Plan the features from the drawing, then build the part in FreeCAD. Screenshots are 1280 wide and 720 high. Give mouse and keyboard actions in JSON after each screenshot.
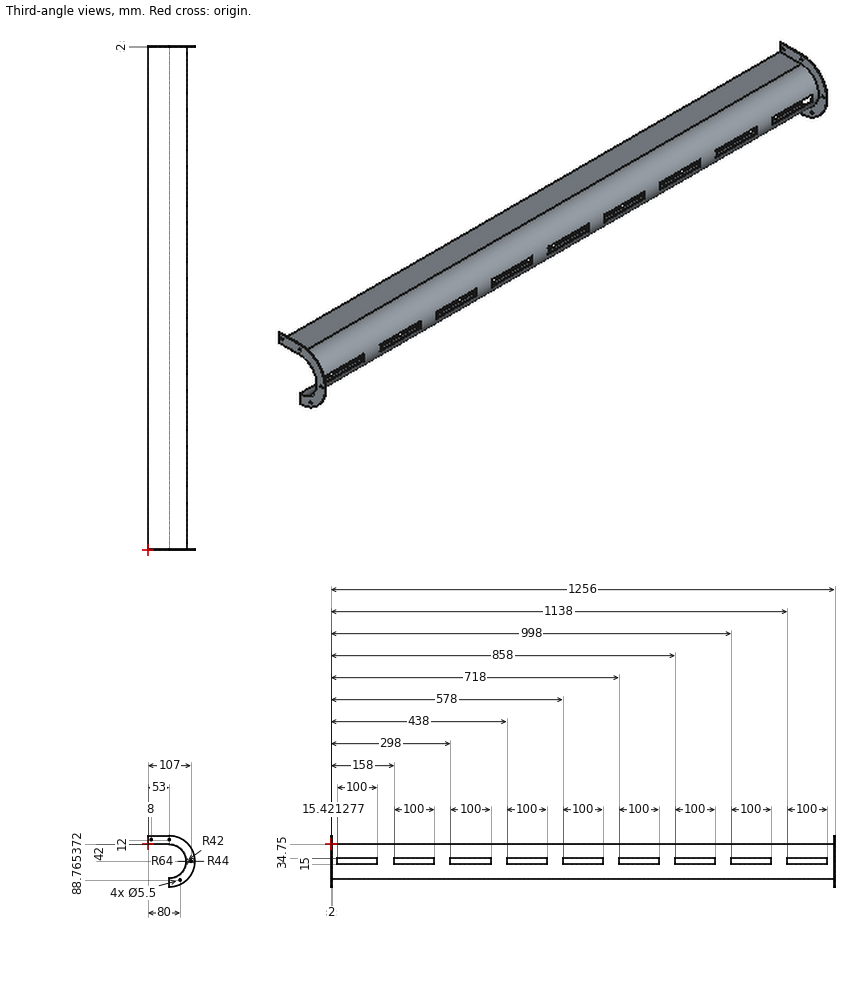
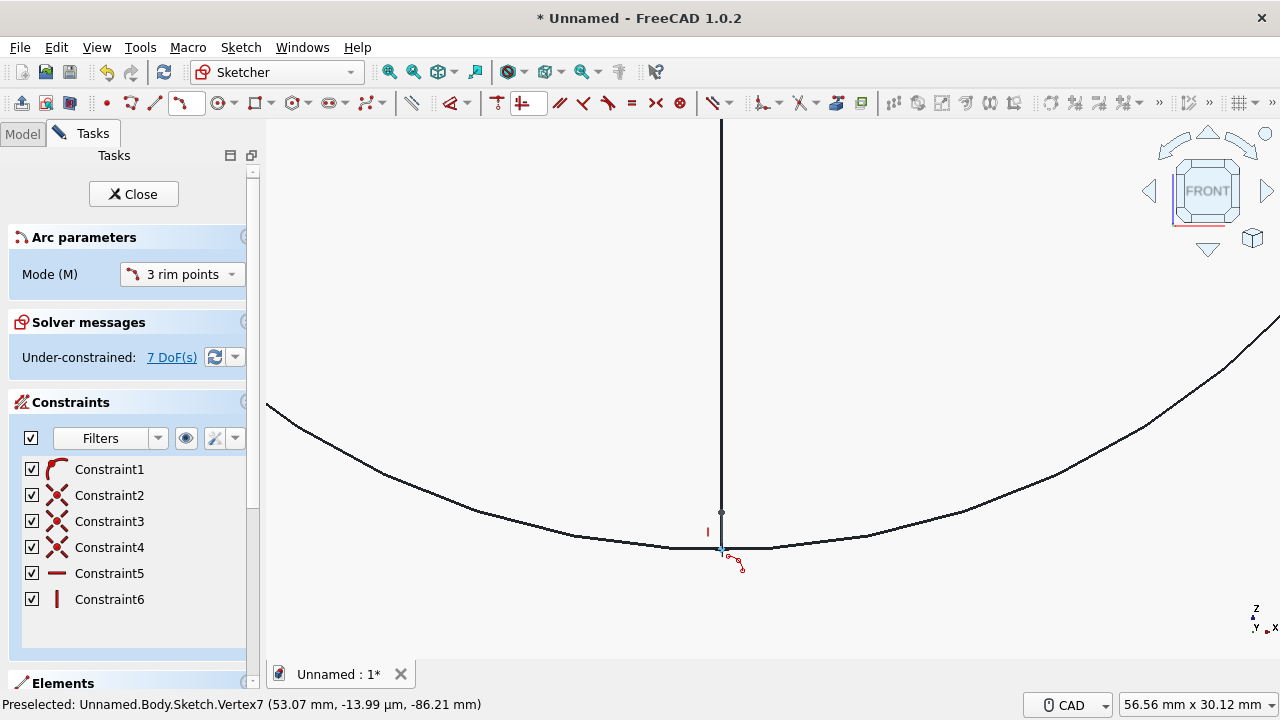
{"action": "scroll", "coordinate": [721, 549], "scroll_direction": "down", "scroll_amount": 8}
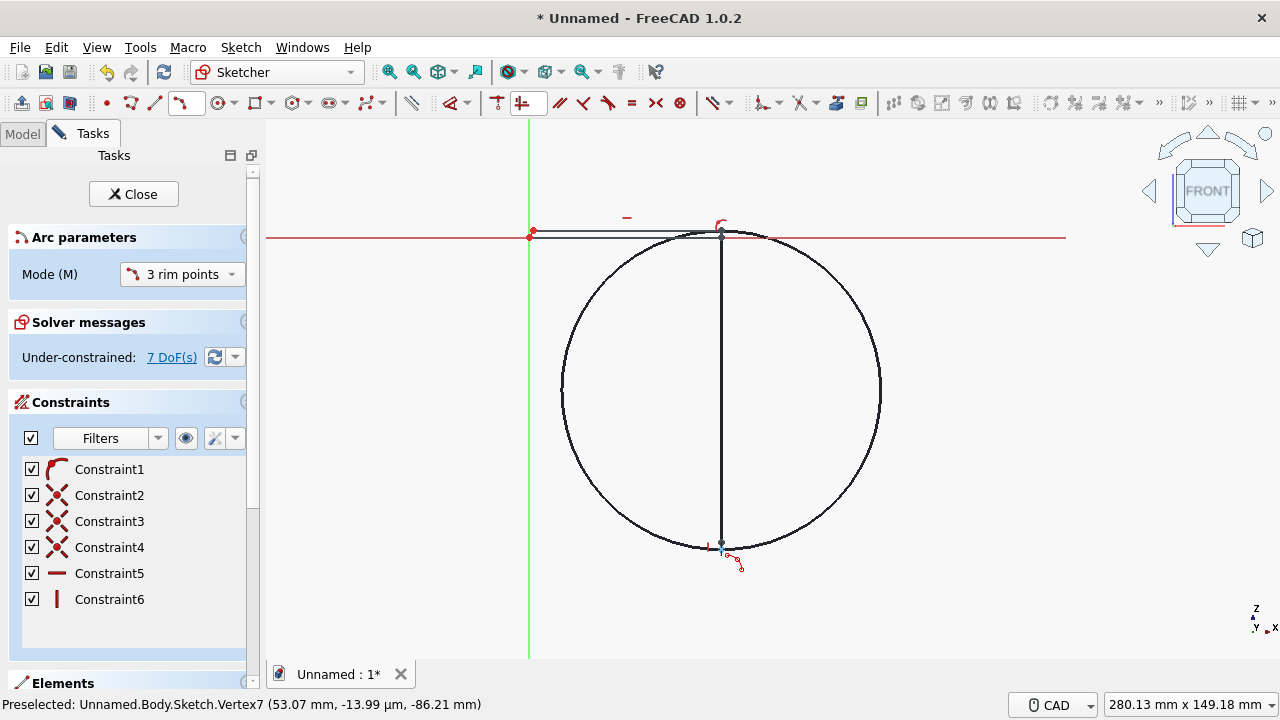
{"action": "left_click", "coordinate": [881, 390]}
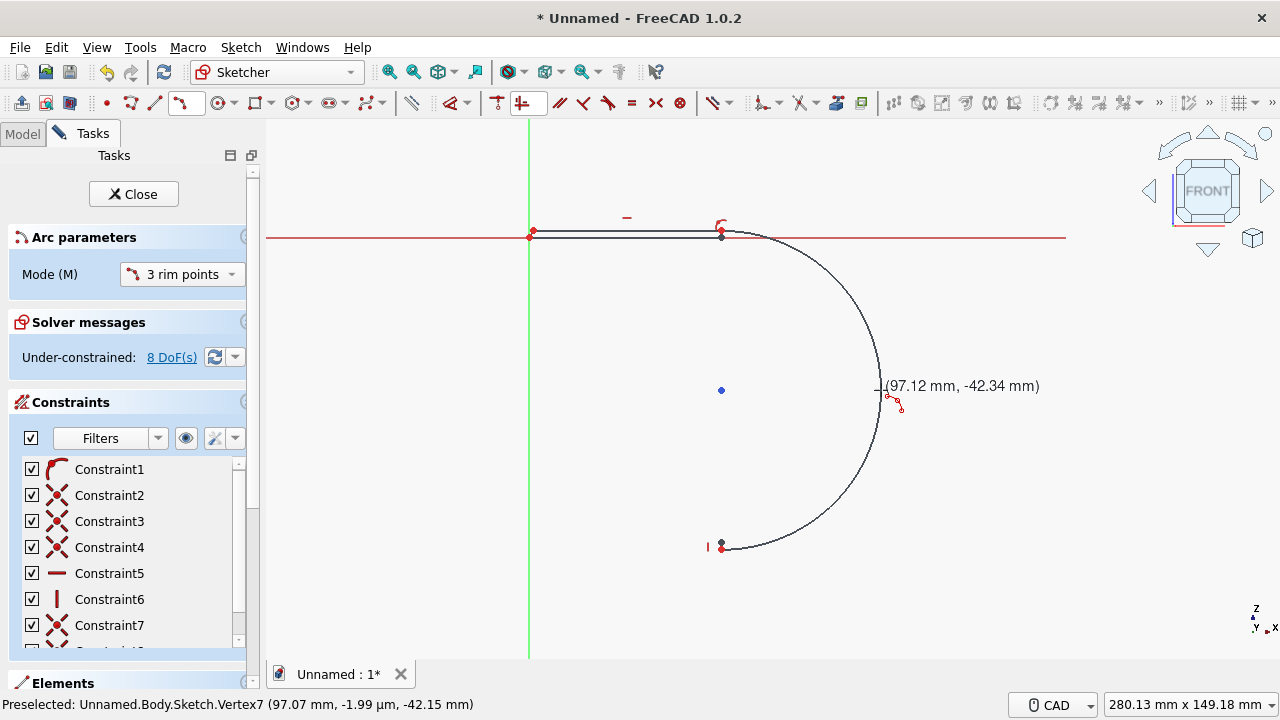
{"action": "scroll", "coordinate": [721, 542], "scroll_direction": "up", "scroll_amount": 8}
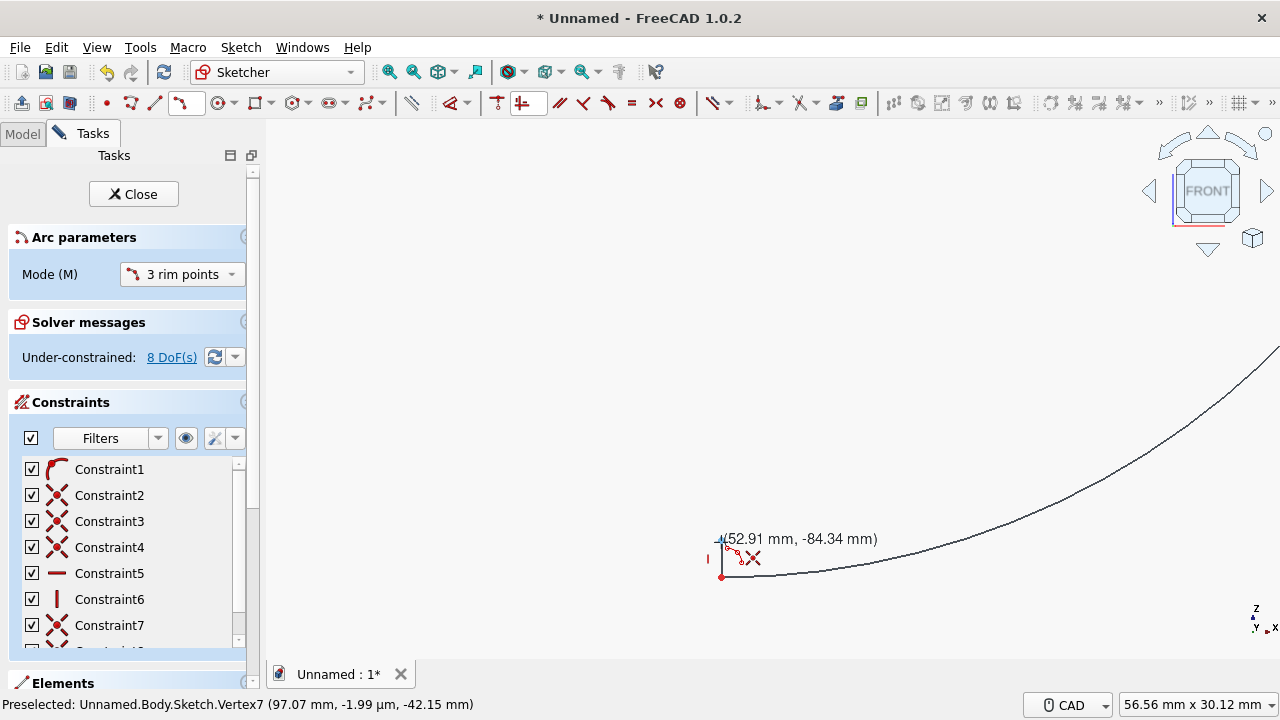
{"action": "left_click", "coordinate": [722, 540]}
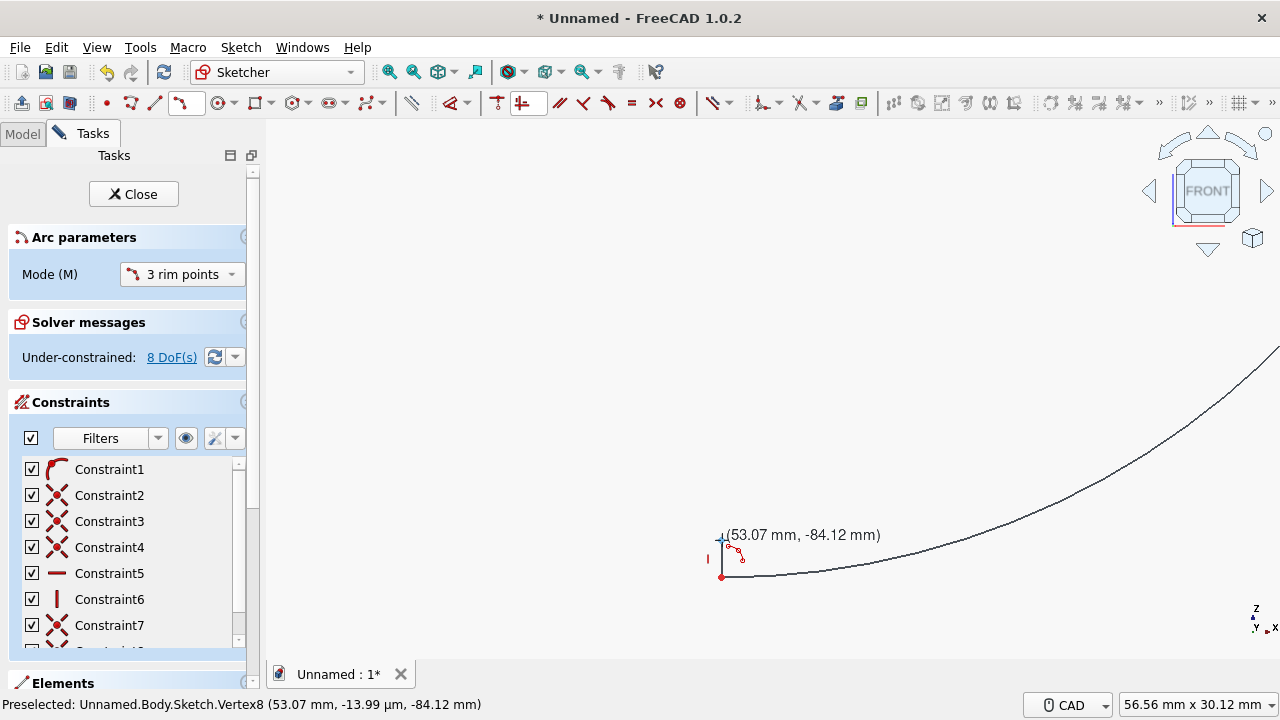
{"action": "scroll", "coordinate": [721, 542], "scroll_direction": "down", "scroll_amount": 8}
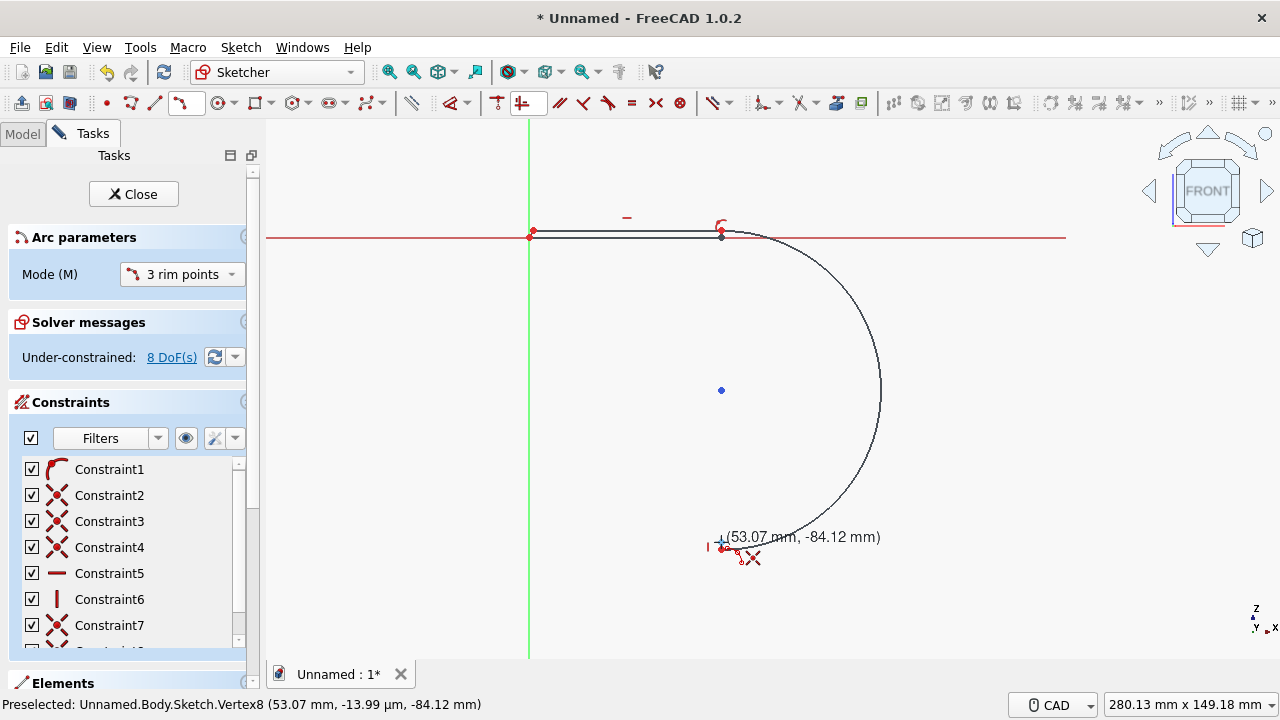
{"action": "scroll", "coordinate": [721, 238], "scroll_direction": "up", "scroll_amount": 4}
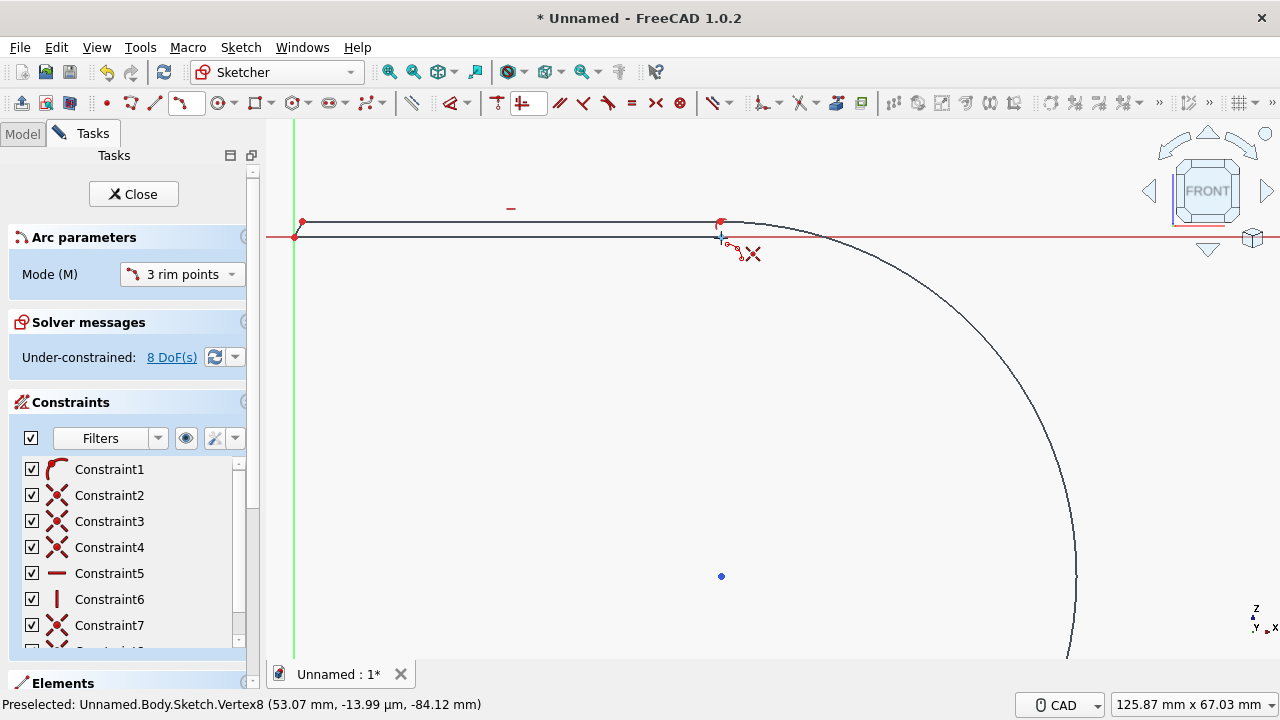
{"action": "left_click", "coordinate": [721, 237]}
{"action": "left_click", "coordinate": [1059, 575]}
{"action": "key", "text": "Escape"}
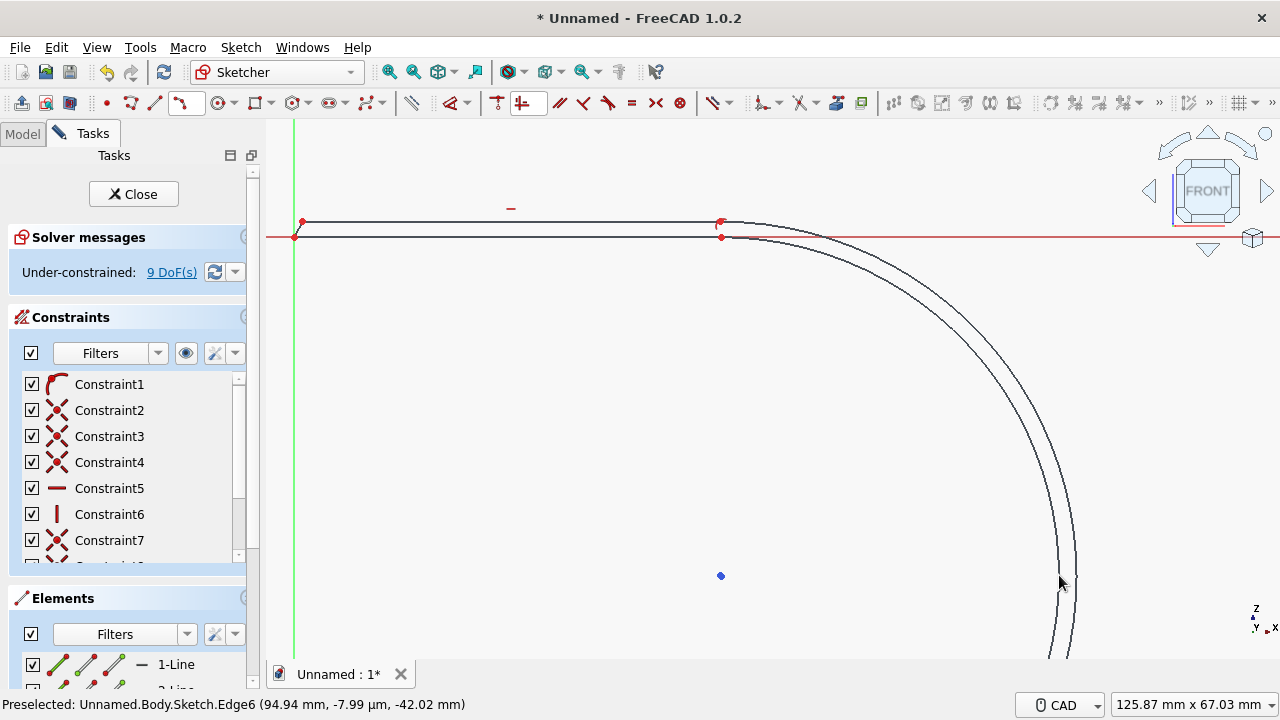
{"action": "scroll", "coordinate": [298, 231], "scroll_direction": "up", "scroll_amount": 5}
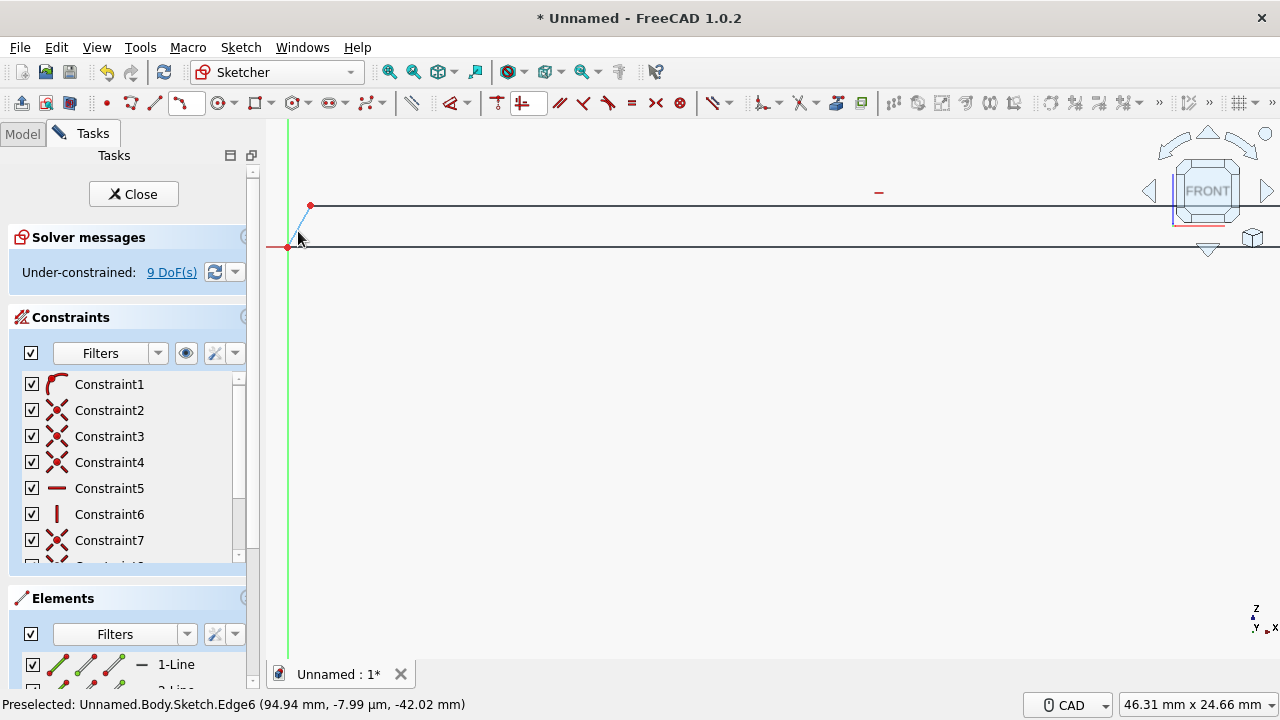
{"action": "left_click", "coordinate": [297, 231]}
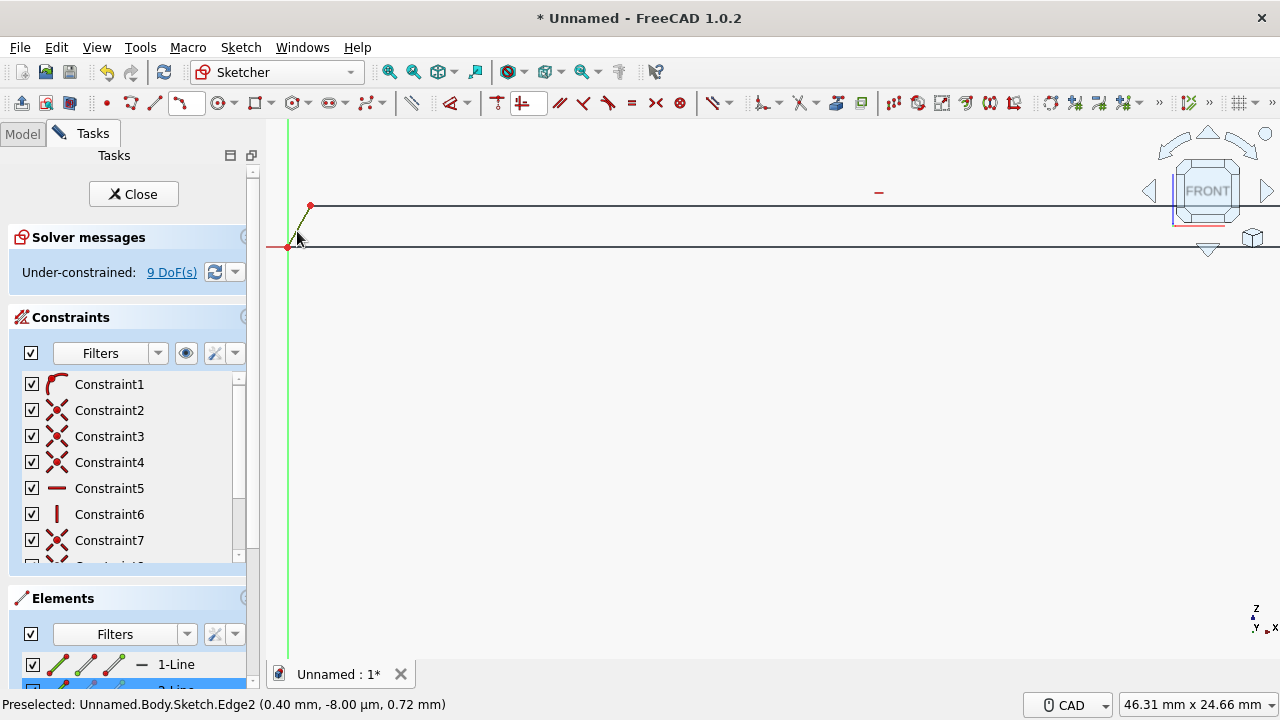
{"action": "key", "text": "v"}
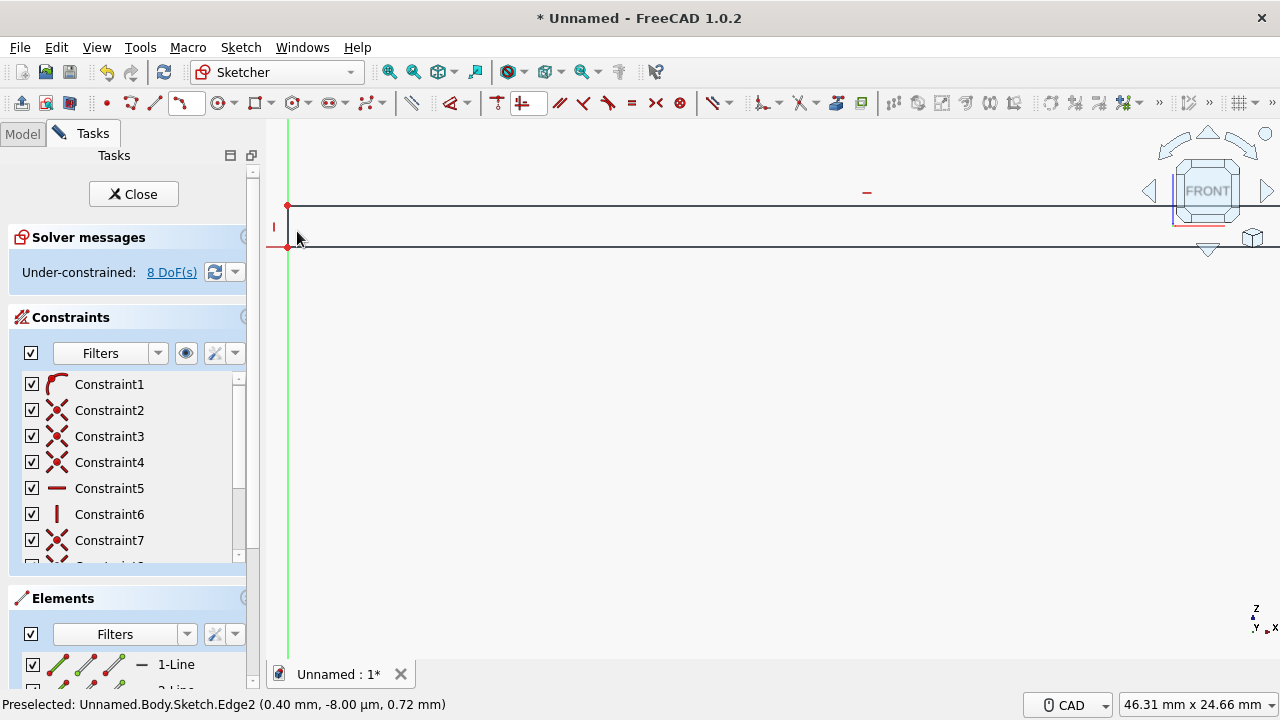
{"action": "scroll", "coordinate": [577, 235], "scroll_direction": "down", "scroll_amount": 9}